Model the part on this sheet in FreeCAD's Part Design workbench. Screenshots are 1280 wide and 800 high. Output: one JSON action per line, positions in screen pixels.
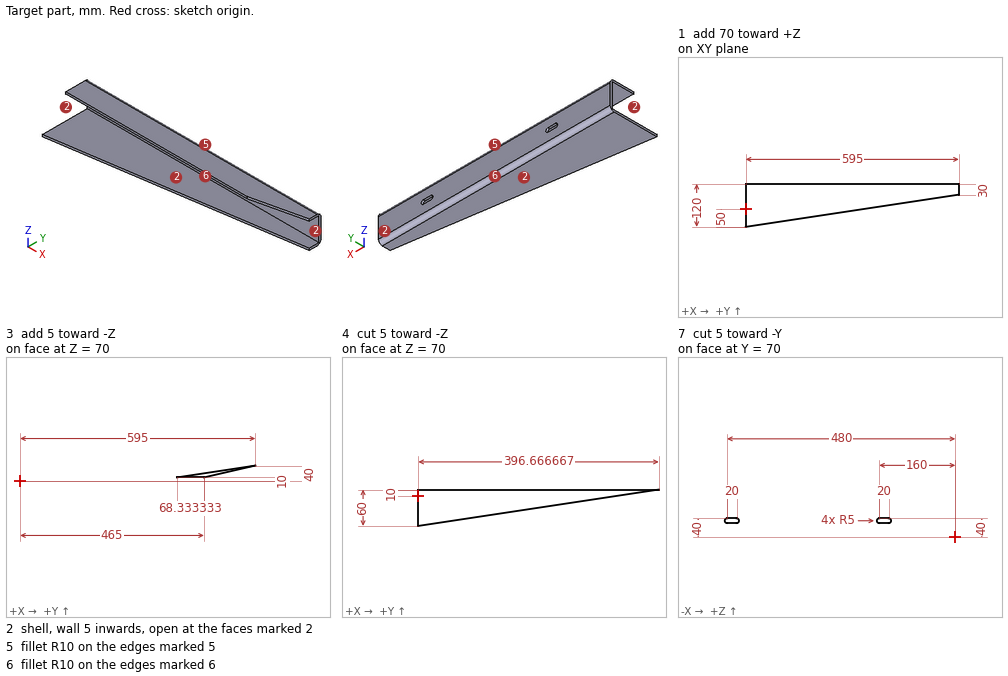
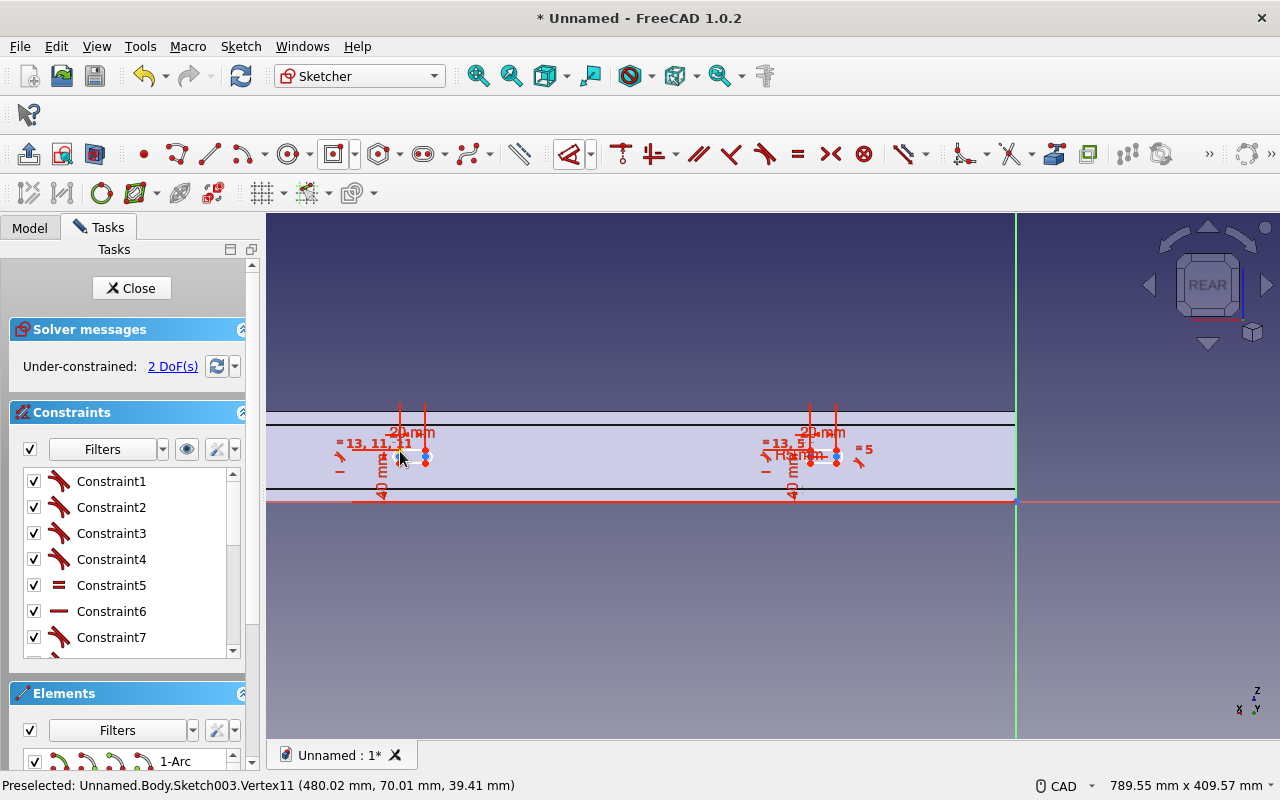
{"action": "scroll", "coordinate": [810, 450], "scroll_direction": "up", "scroll_amount": 4}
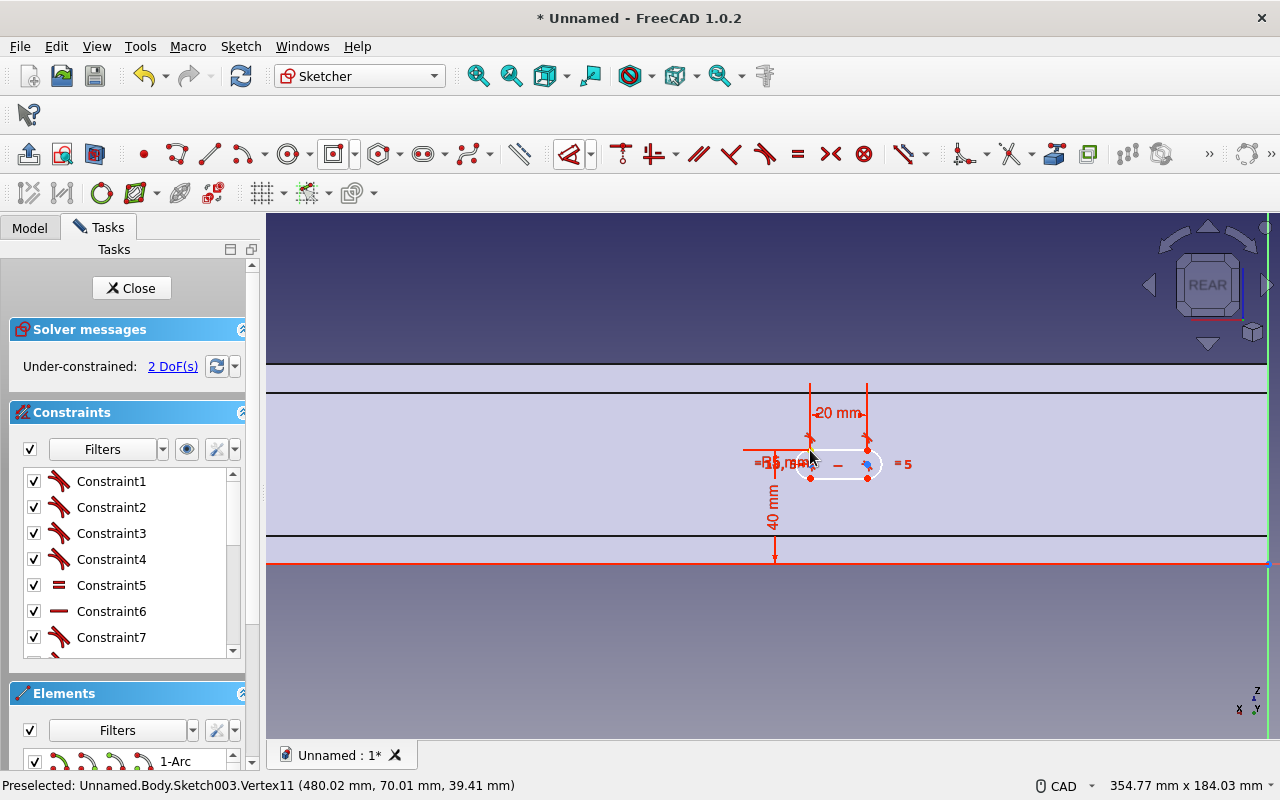
{"action": "left_click", "coordinate": [810, 450]}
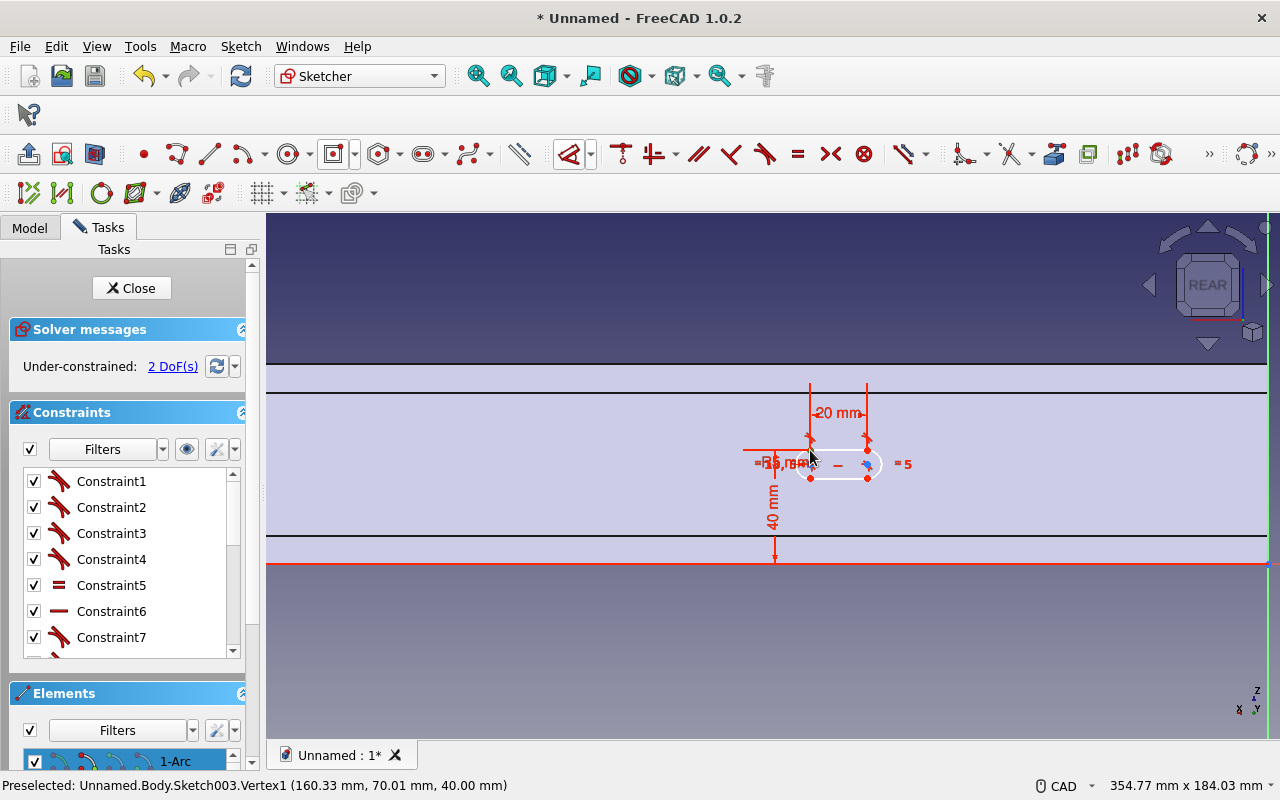
{"action": "left_click", "coordinate": [590, 154]}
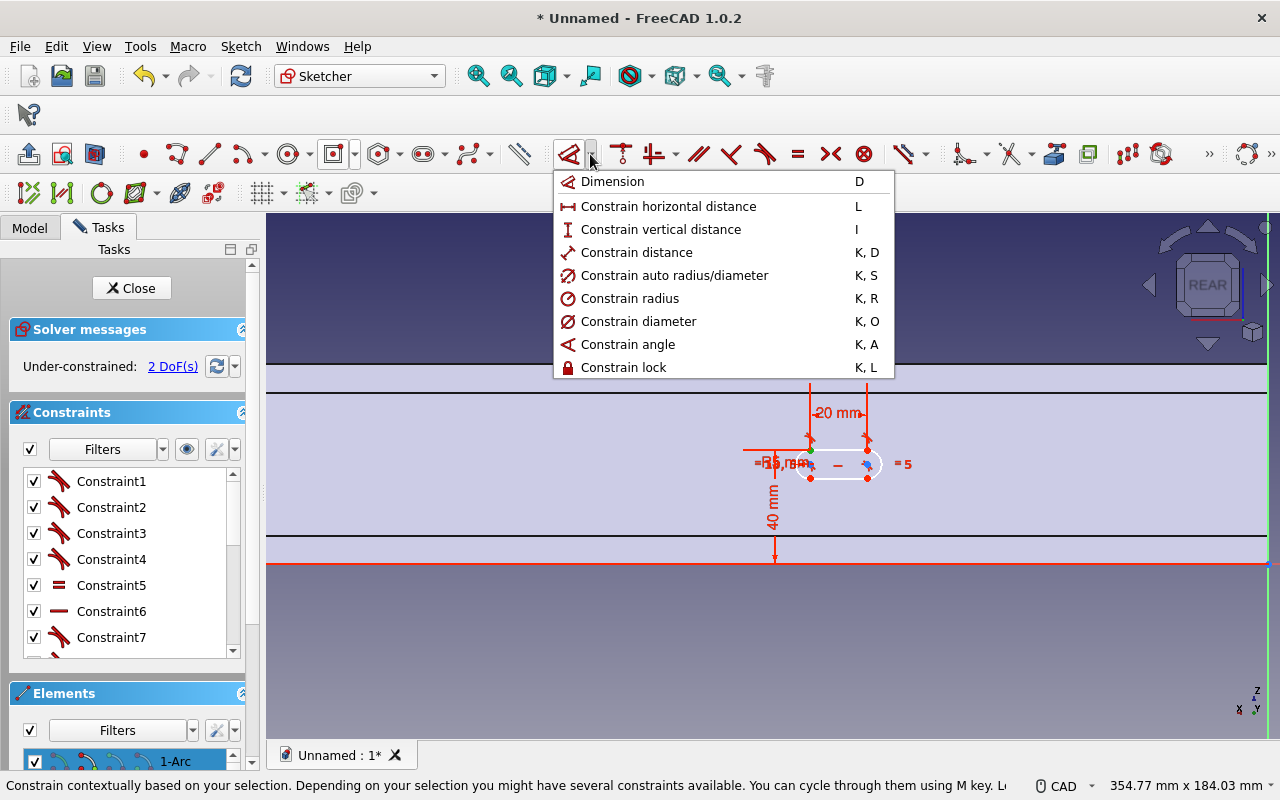
{"action": "left_click", "coordinate": [724, 206]}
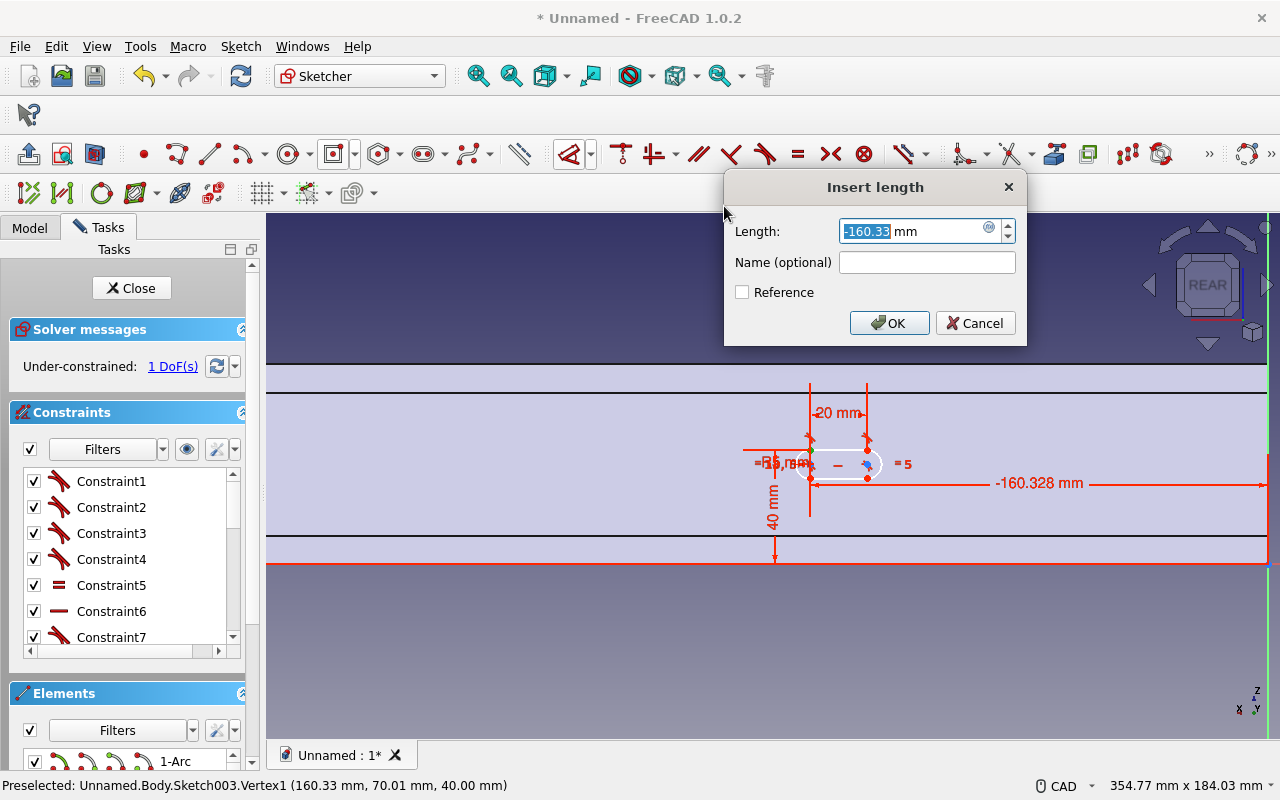
{"action": "type", "text": "-160"}
{"action": "key", "text": "Return"}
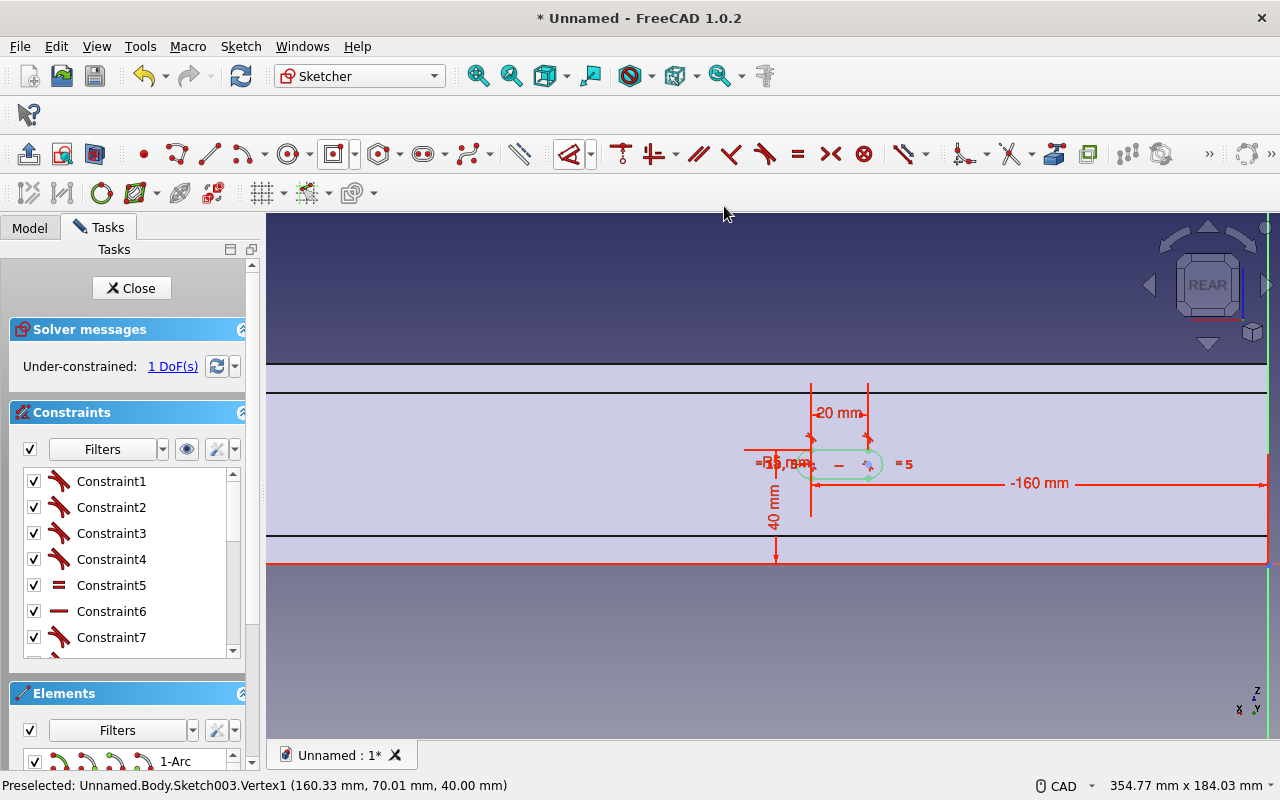
{"action": "scroll", "coordinate": [810, 450], "scroll_direction": "down", "scroll_amount": 4}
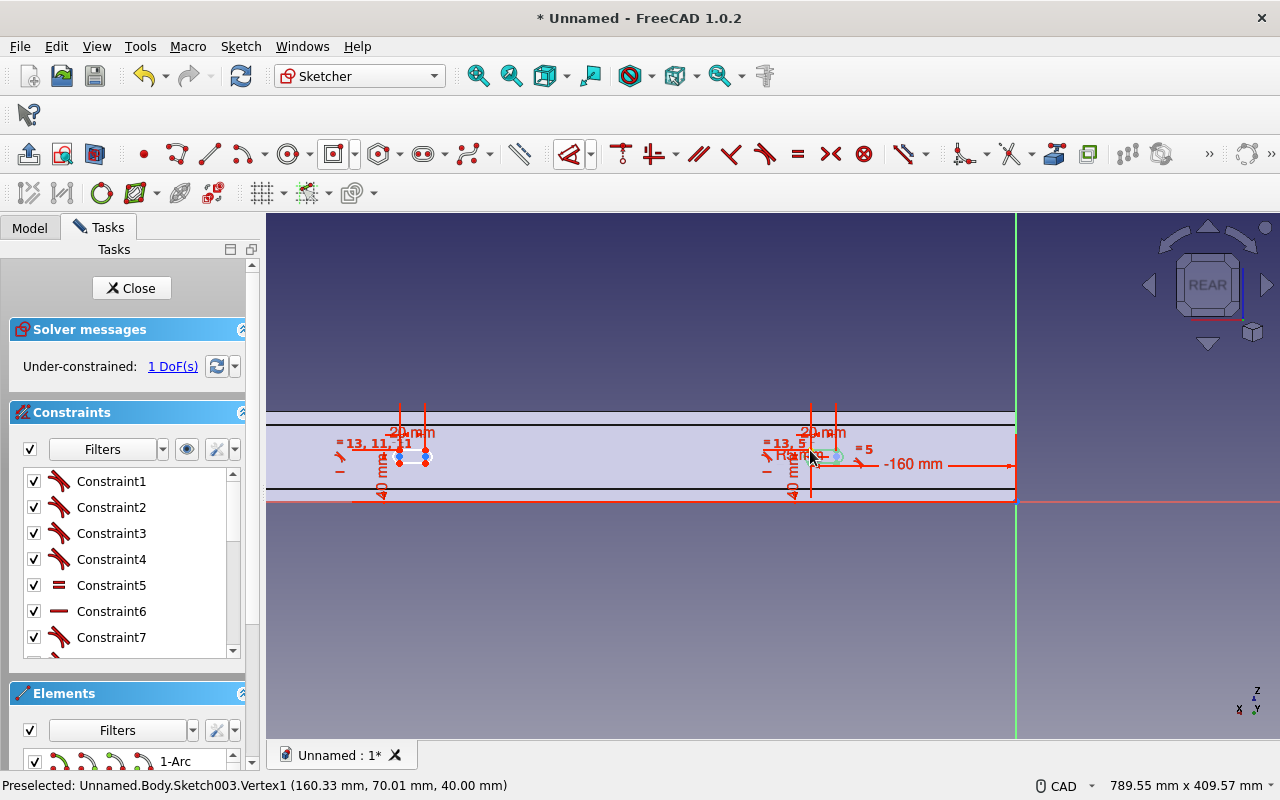
{"action": "scroll", "coordinate": [400, 450], "scroll_direction": "up", "scroll_amount": 4}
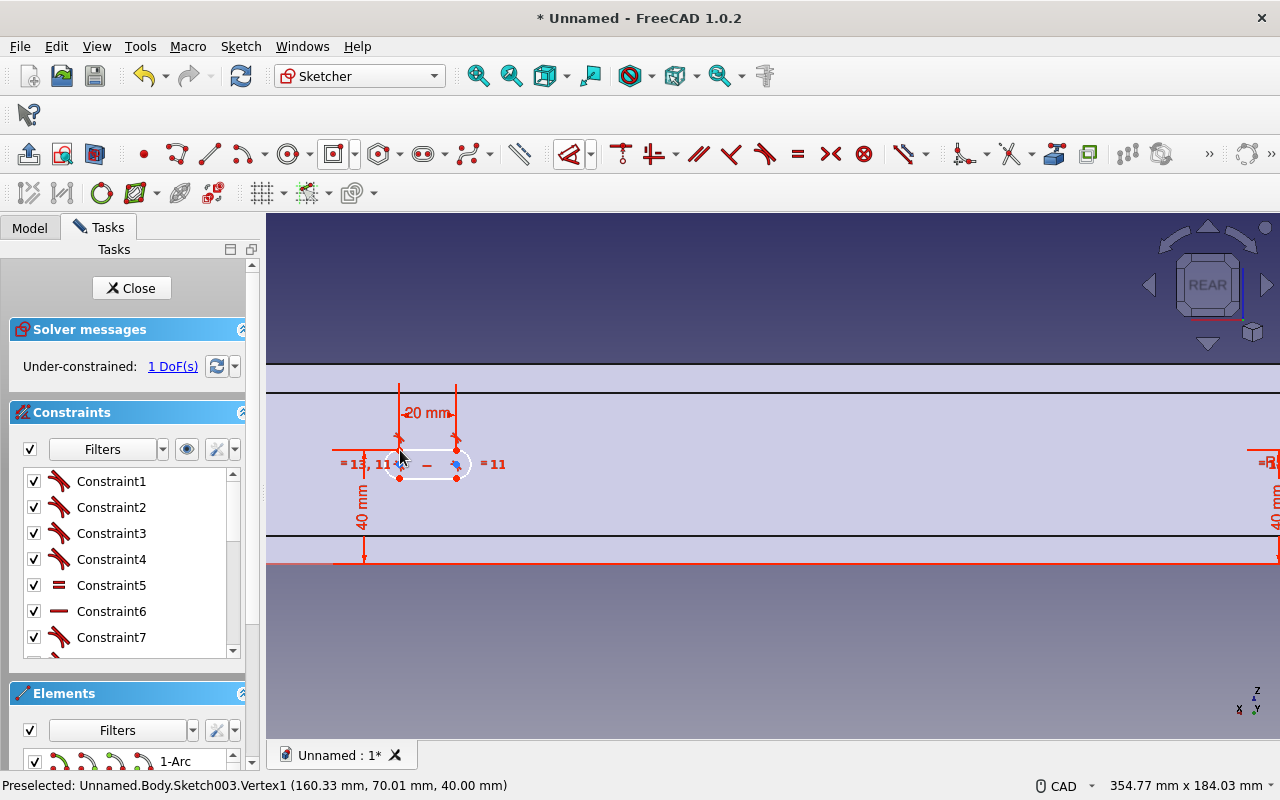
{"action": "left_click", "coordinate": [399, 450]}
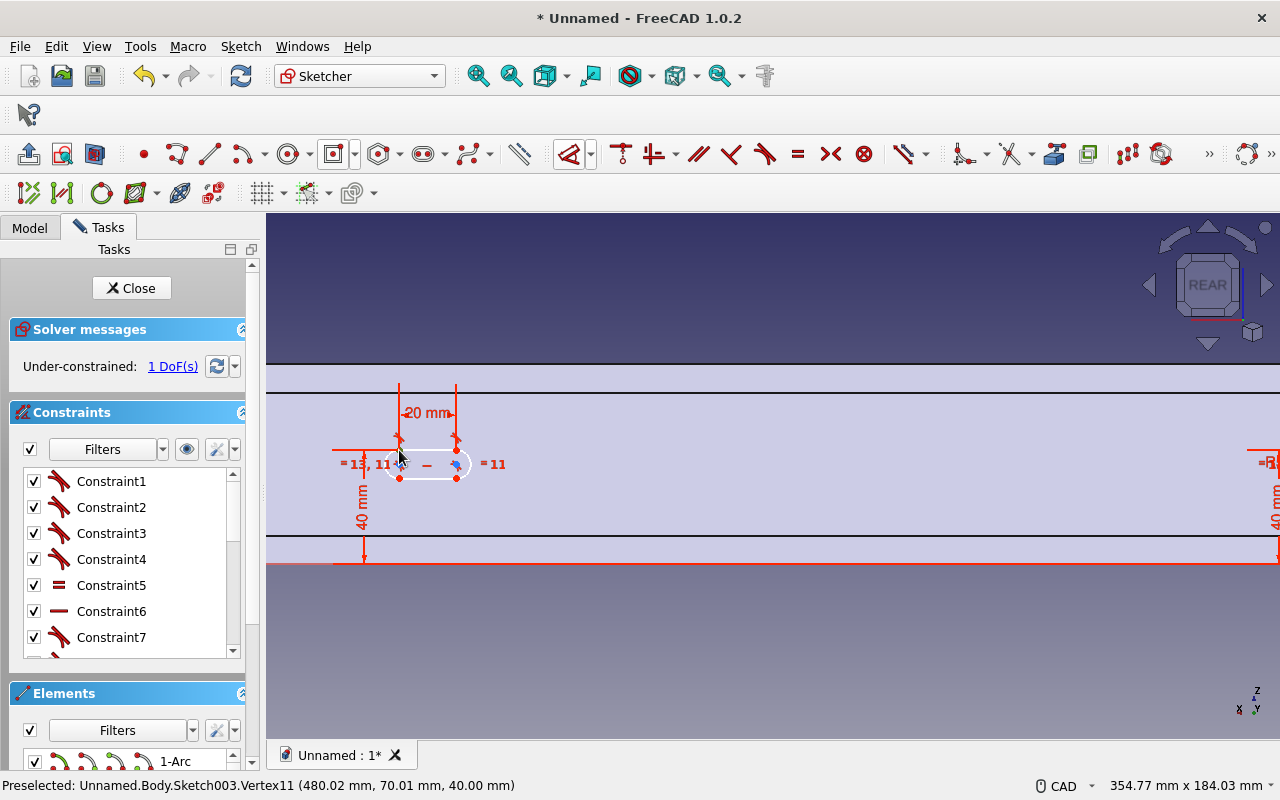
{"action": "key", "text": "l"}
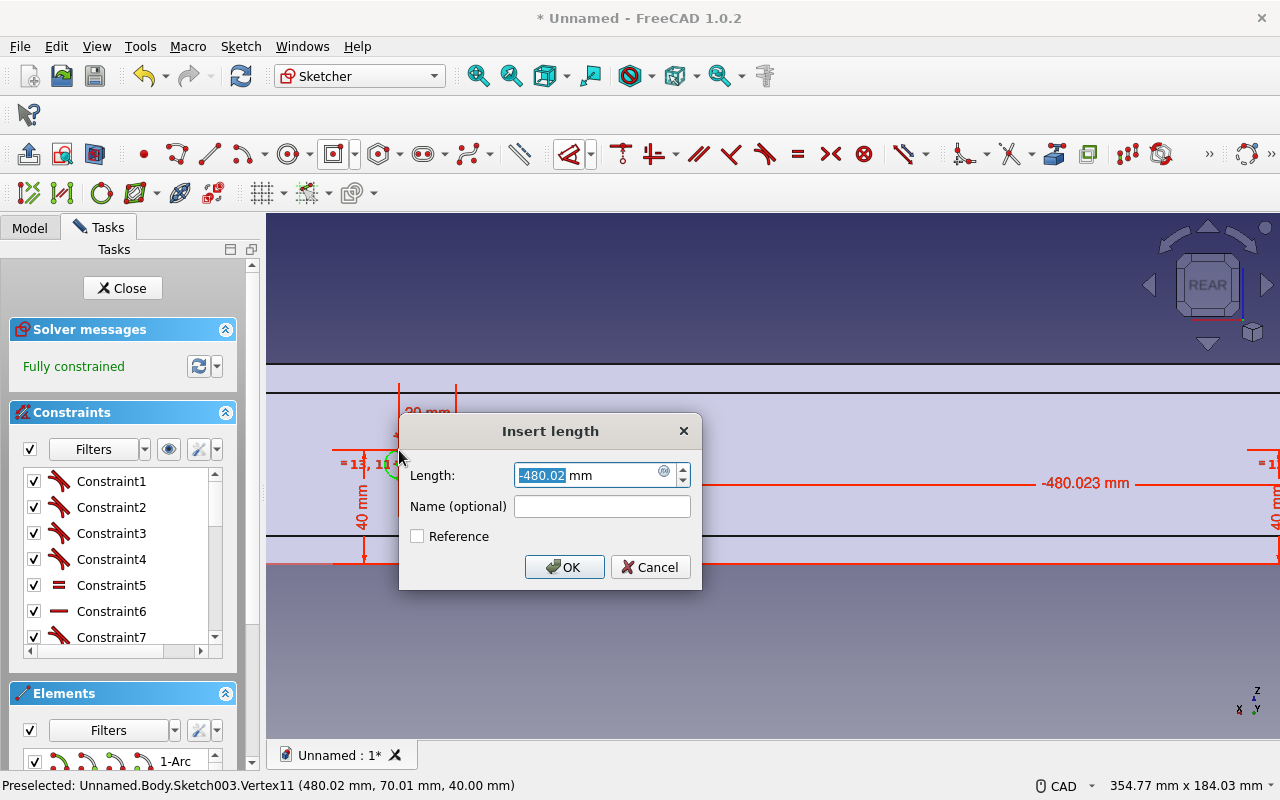
{"action": "type", "text": "-480"}
{"action": "key", "text": "Return"}